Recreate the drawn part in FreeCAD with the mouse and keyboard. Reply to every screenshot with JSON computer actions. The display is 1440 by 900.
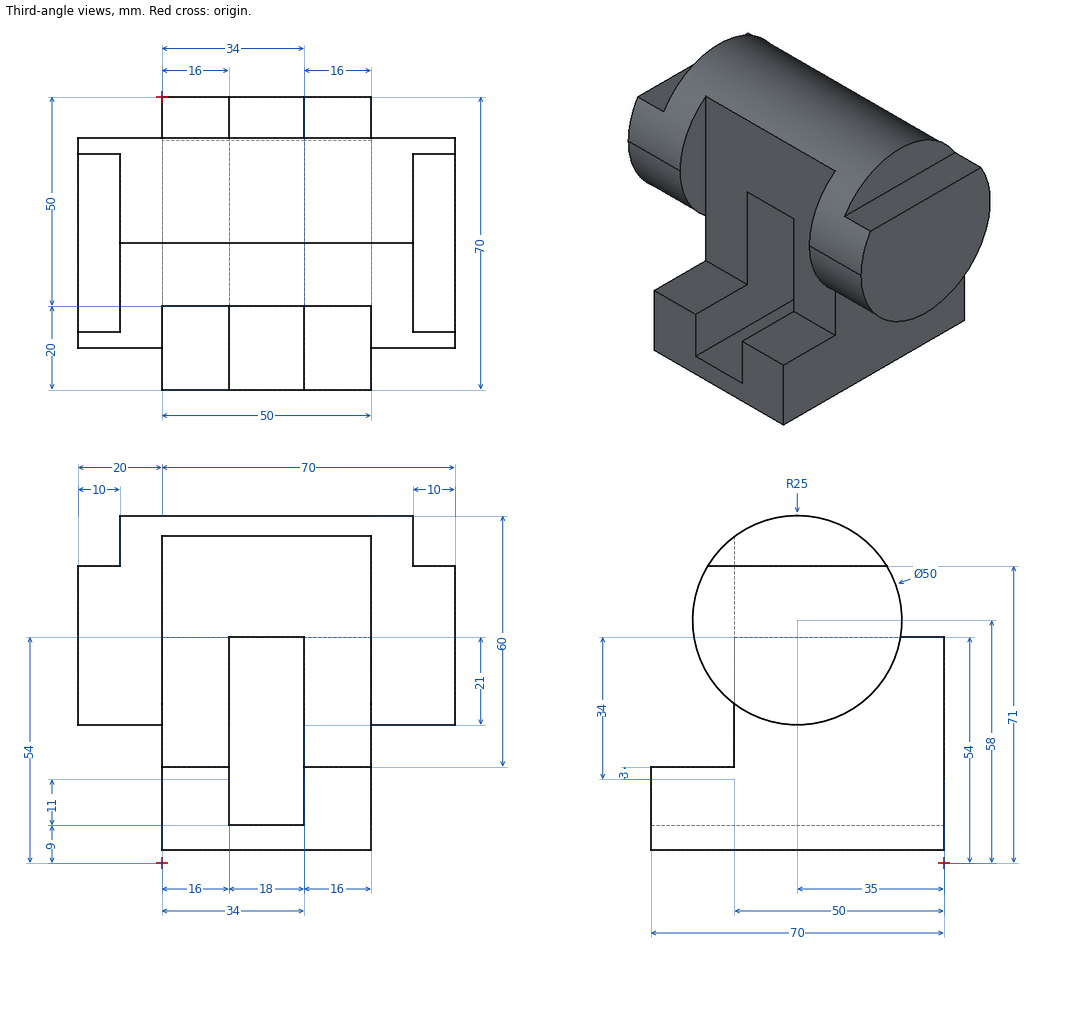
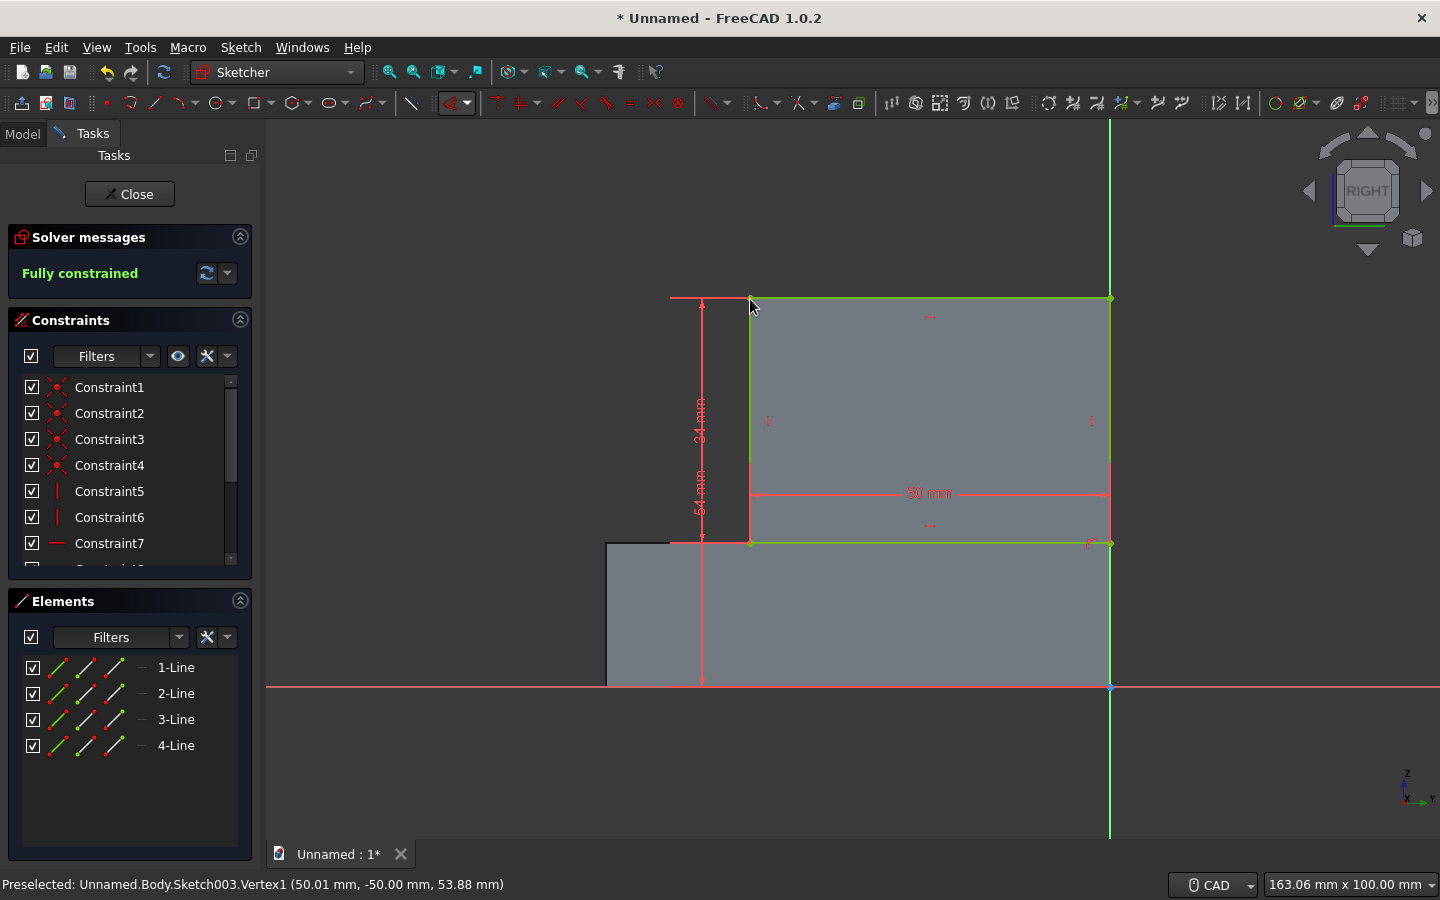
{"action": "left_click", "coordinate": [130, 194]}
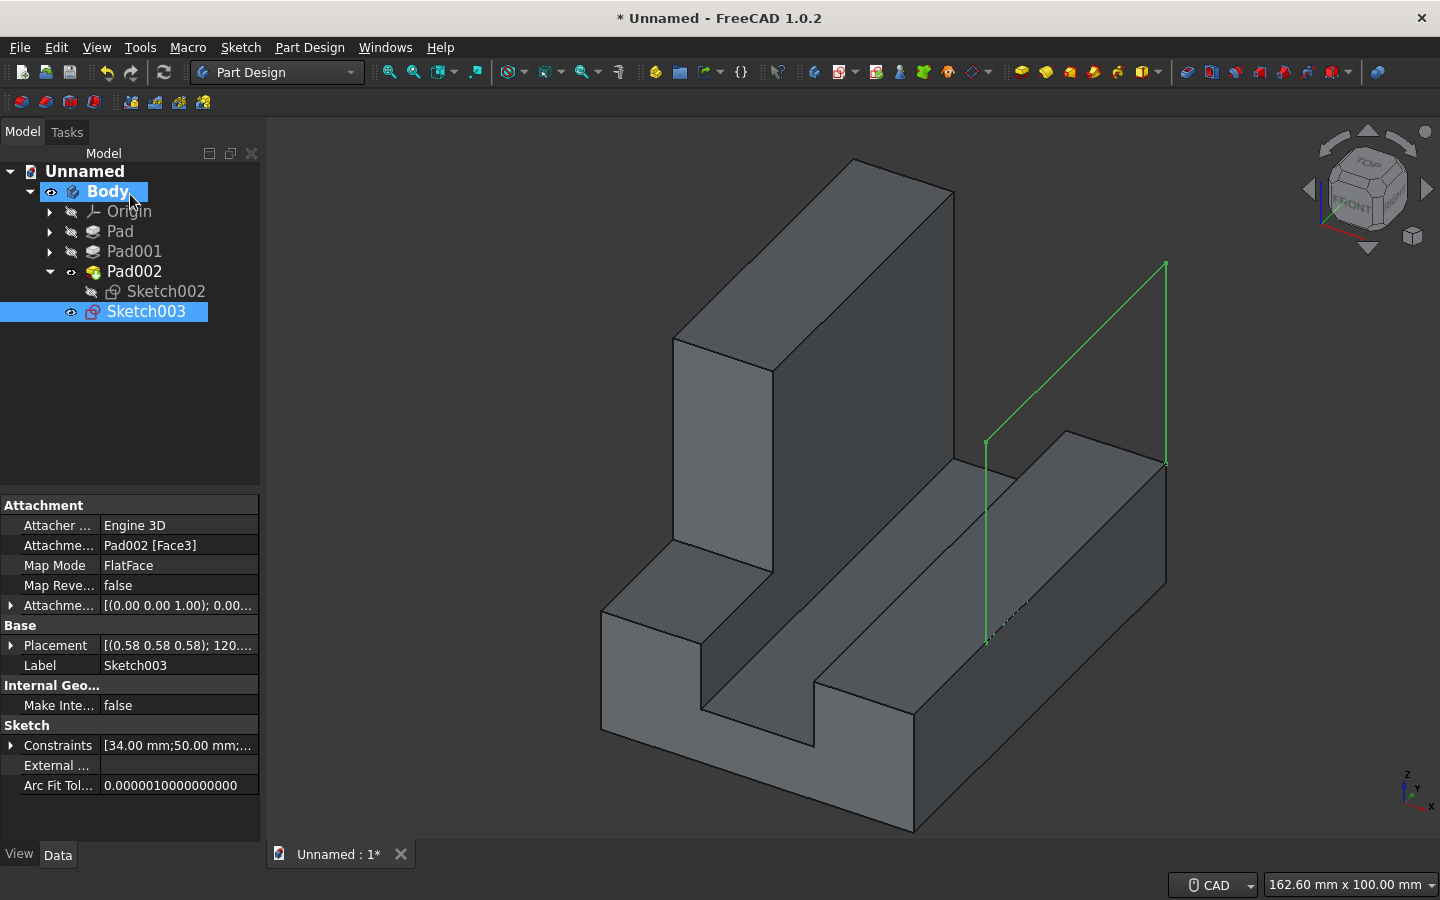
{"action": "left_click", "coordinate": [1022, 72]}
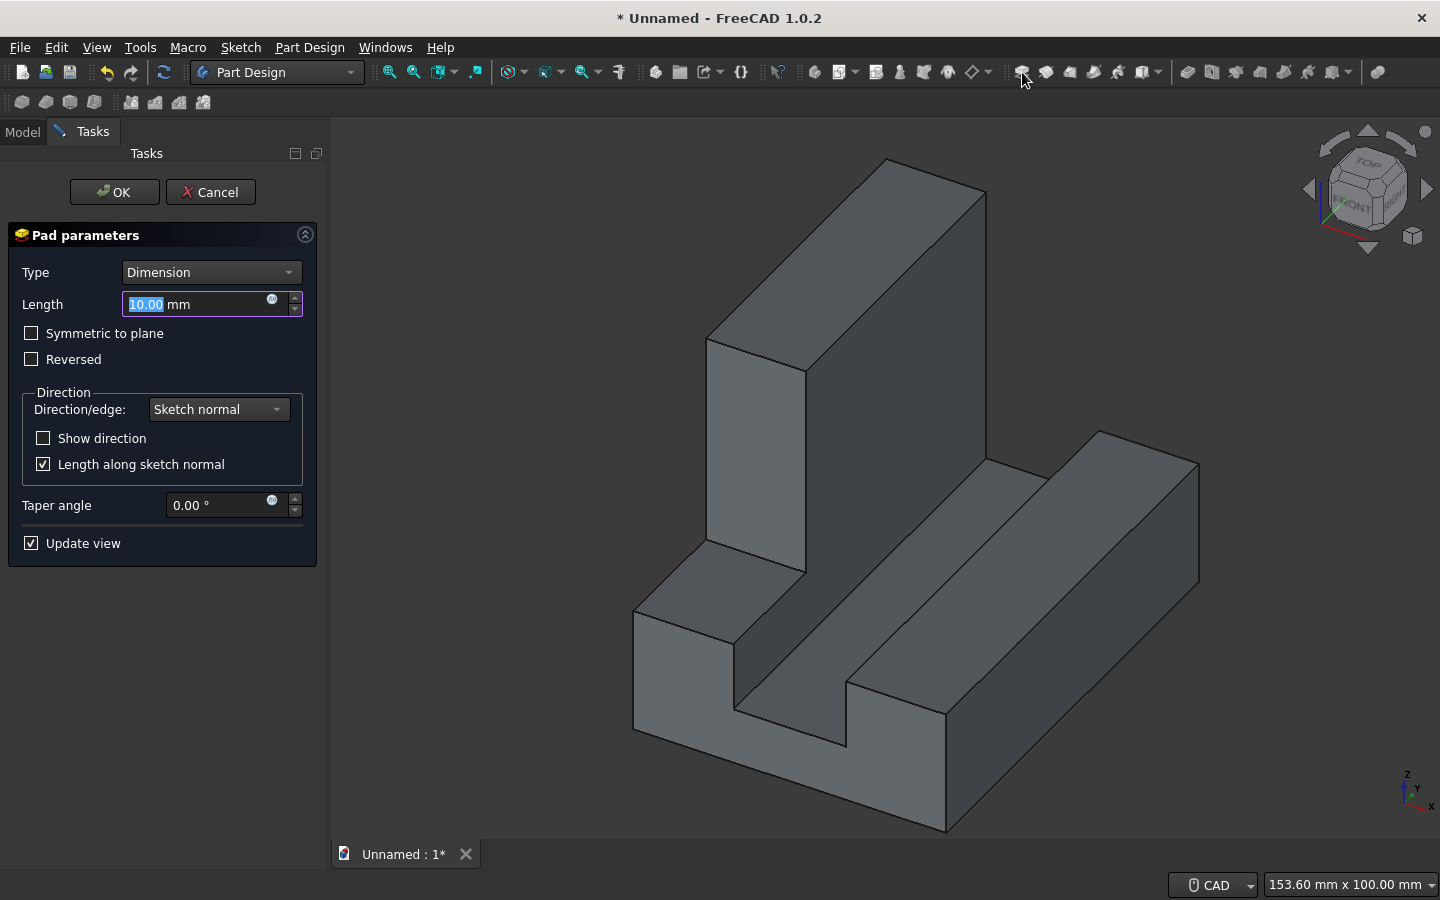
{"action": "type", "text": "16"}
{"action": "key", "text": "Tab"}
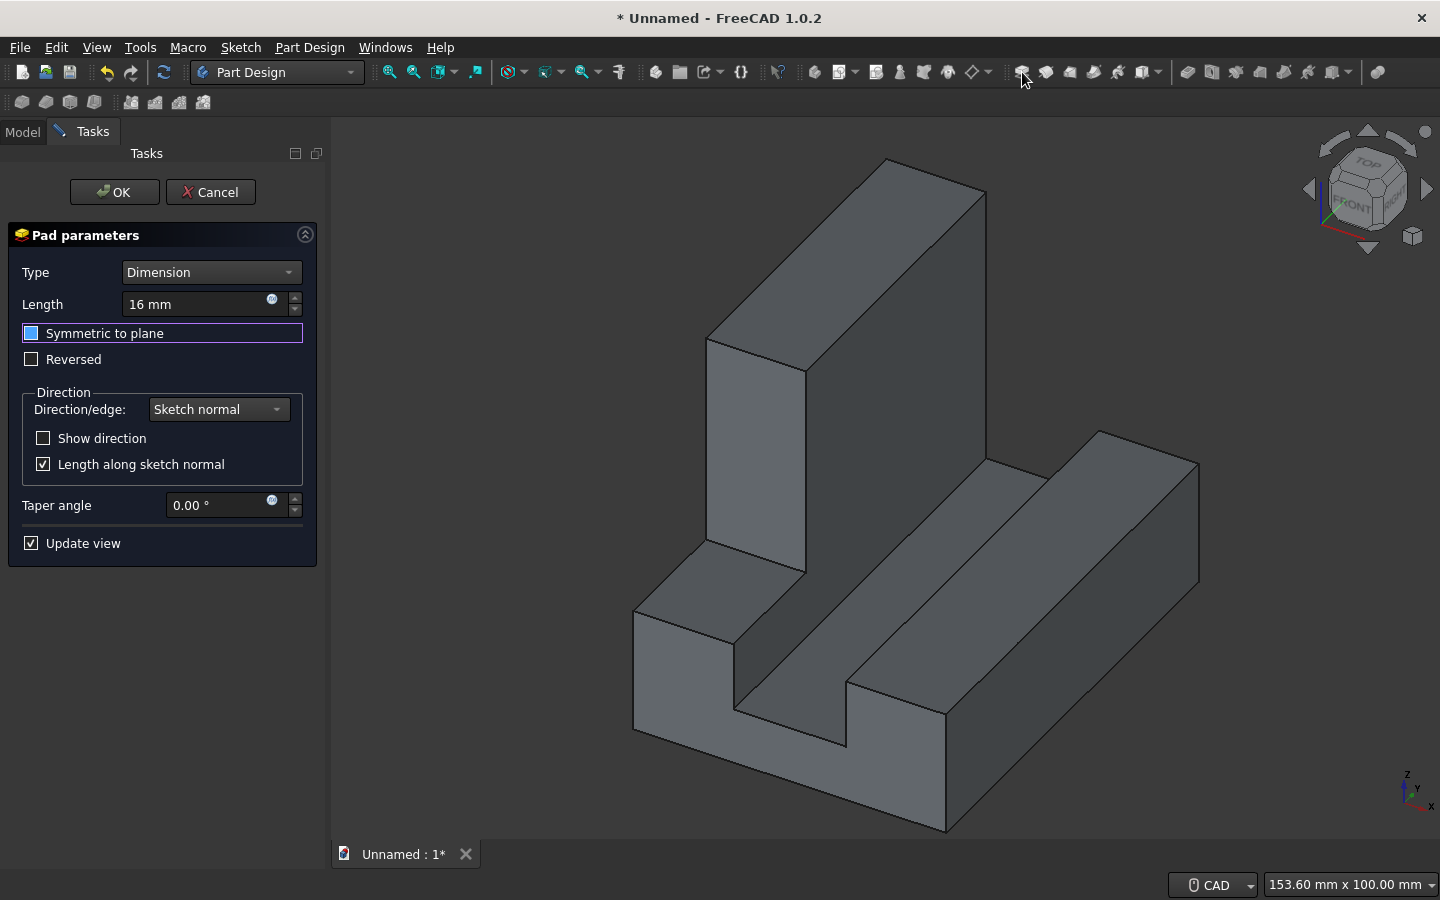
{"action": "left_click", "coordinate": [30, 359]}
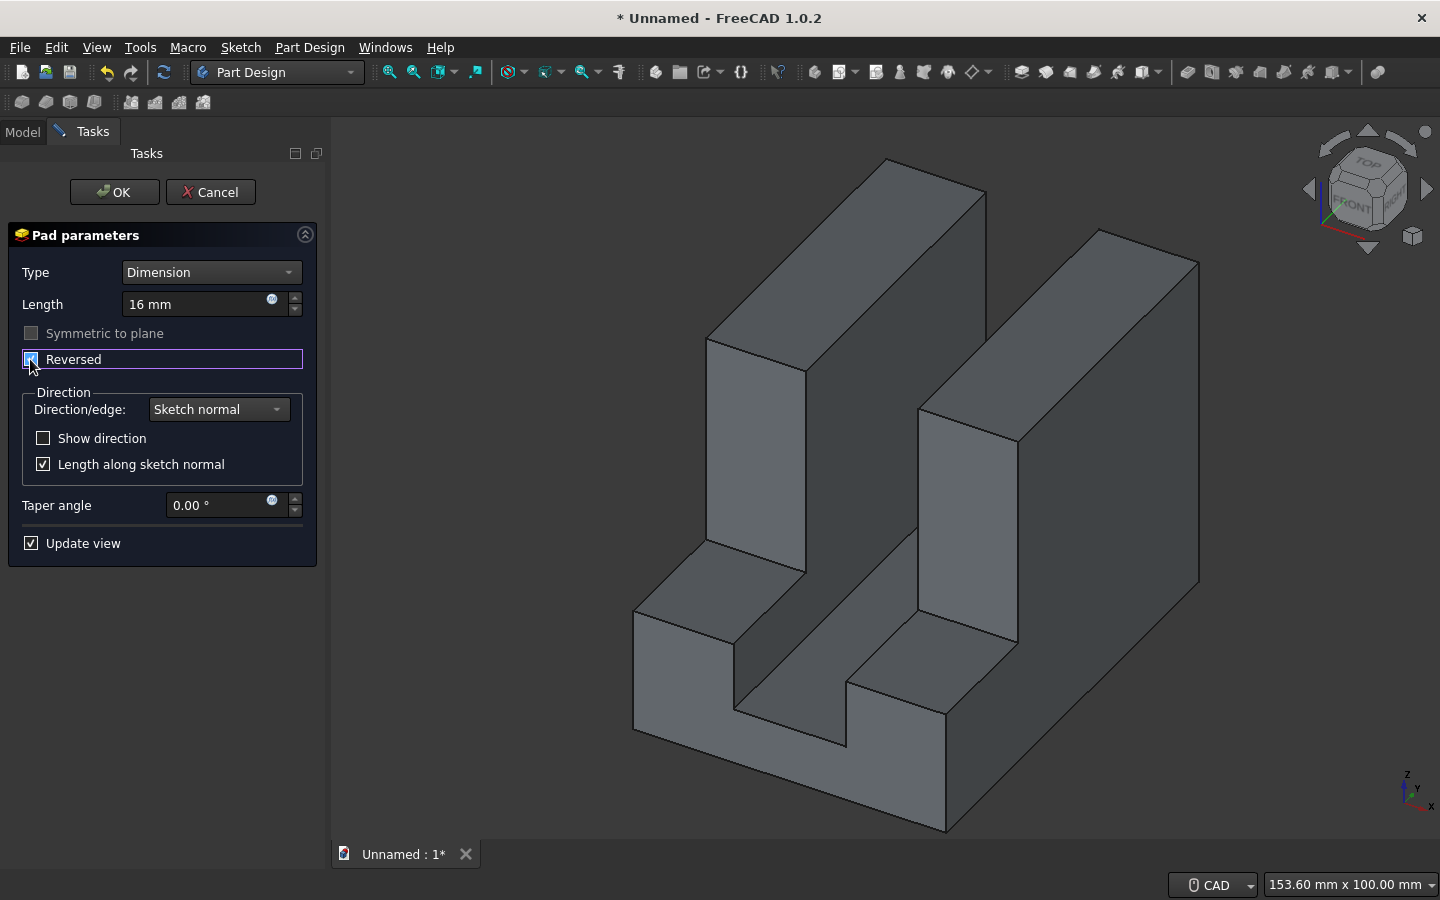
{"action": "left_click", "coordinate": [115, 192]}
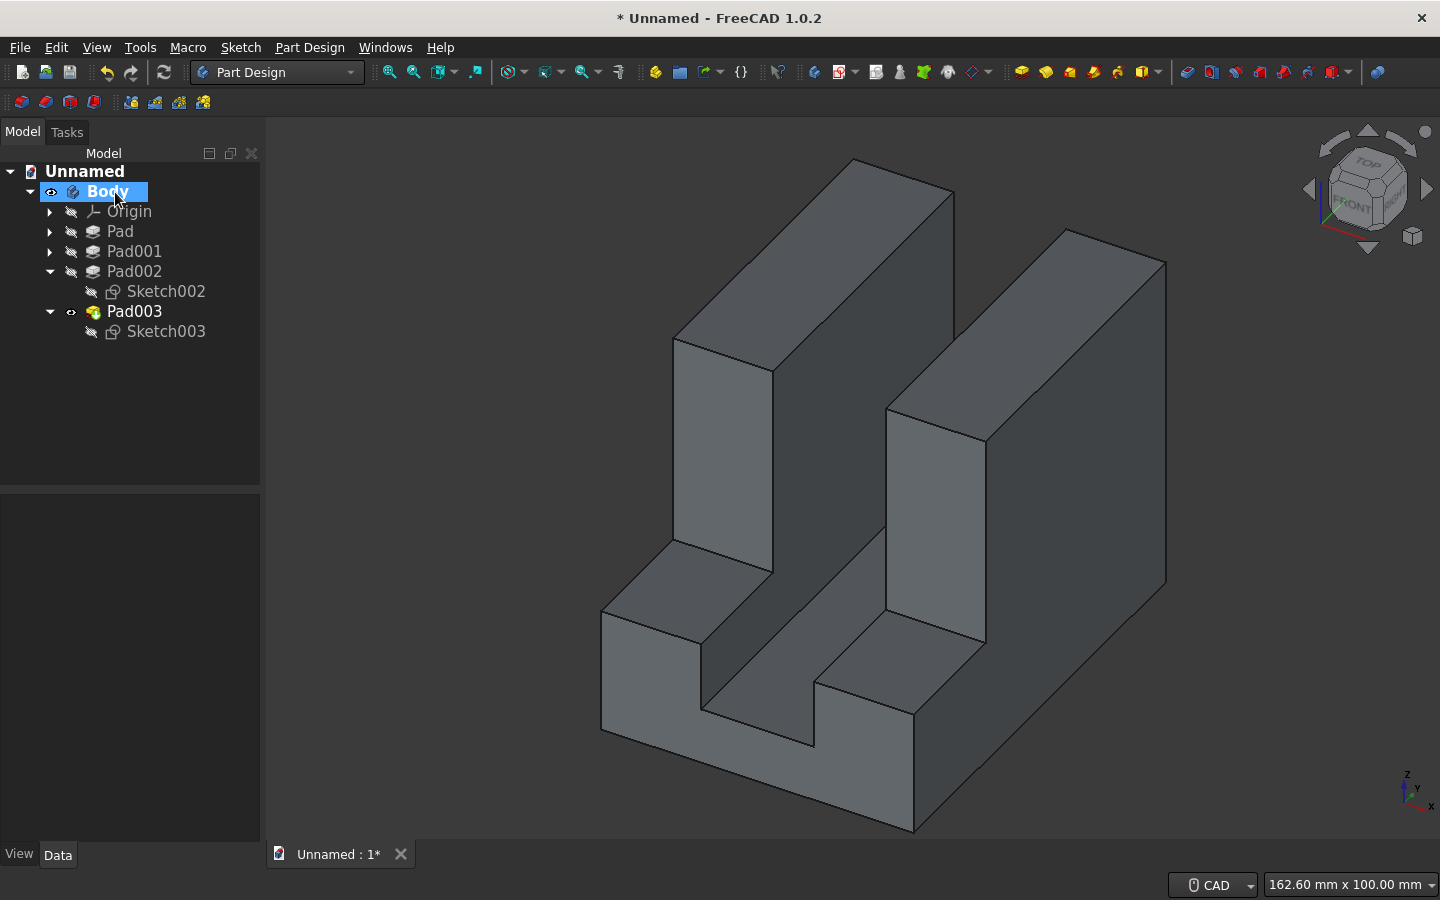
{"action": "key", "text": "5"}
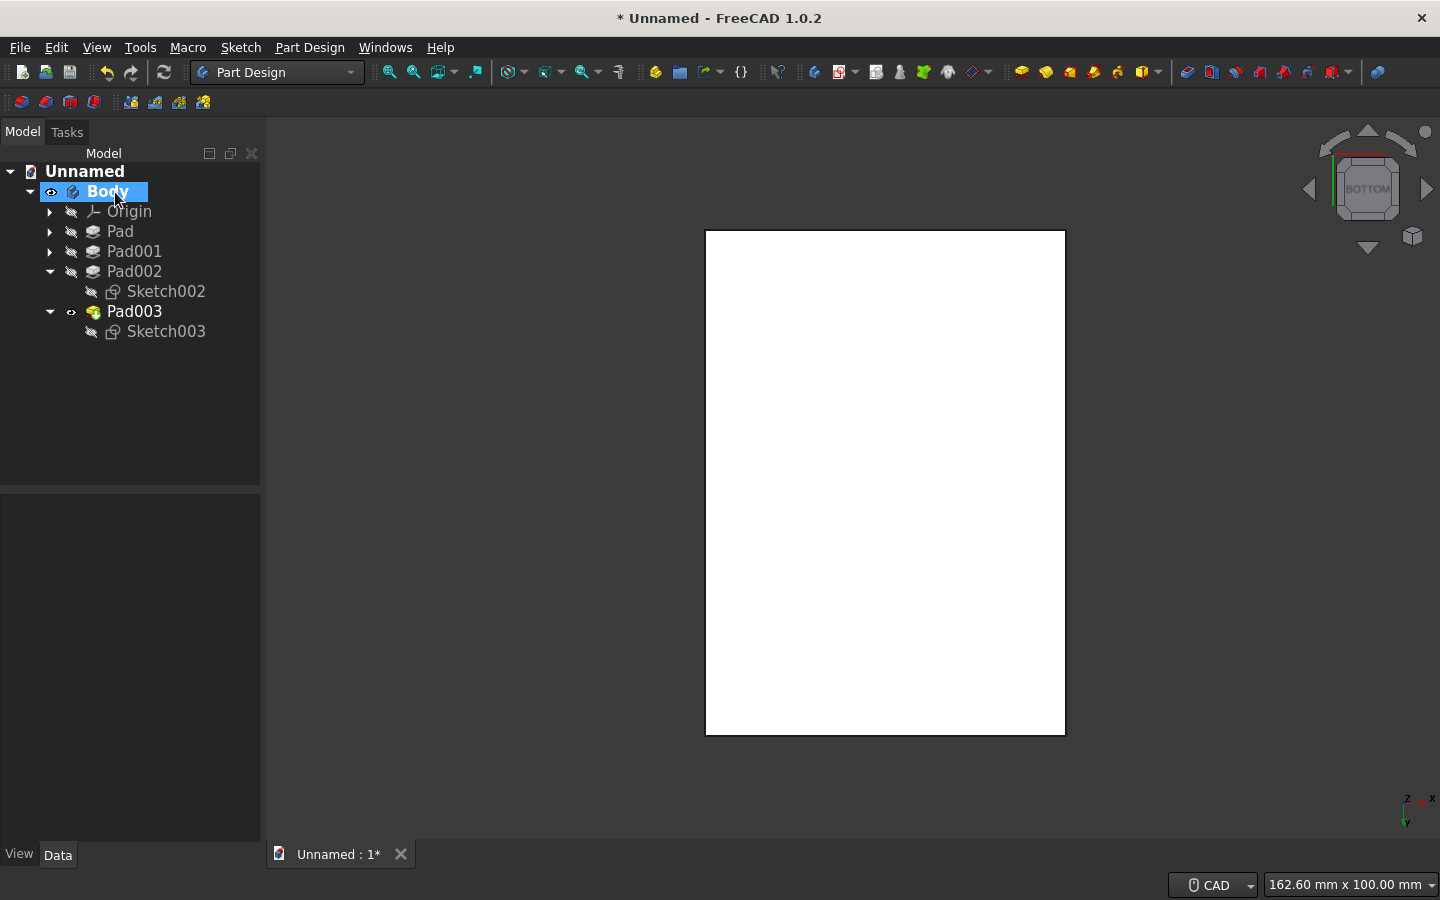
{"action": "left_click", "coordinate": [885, 554]}